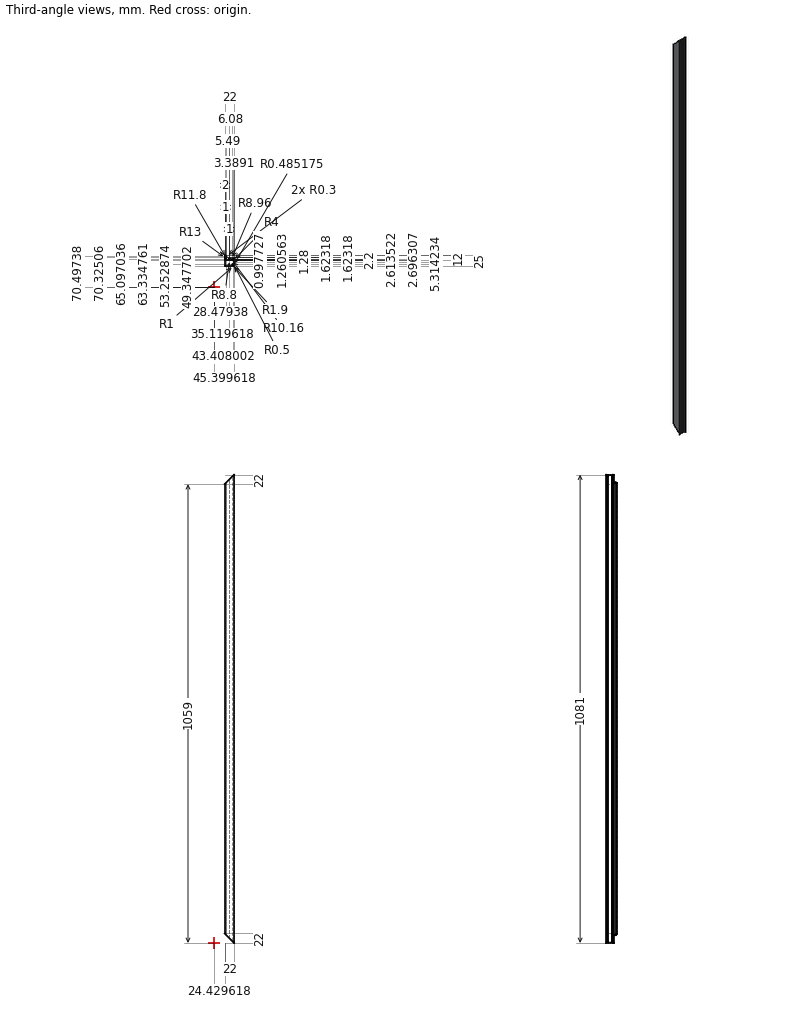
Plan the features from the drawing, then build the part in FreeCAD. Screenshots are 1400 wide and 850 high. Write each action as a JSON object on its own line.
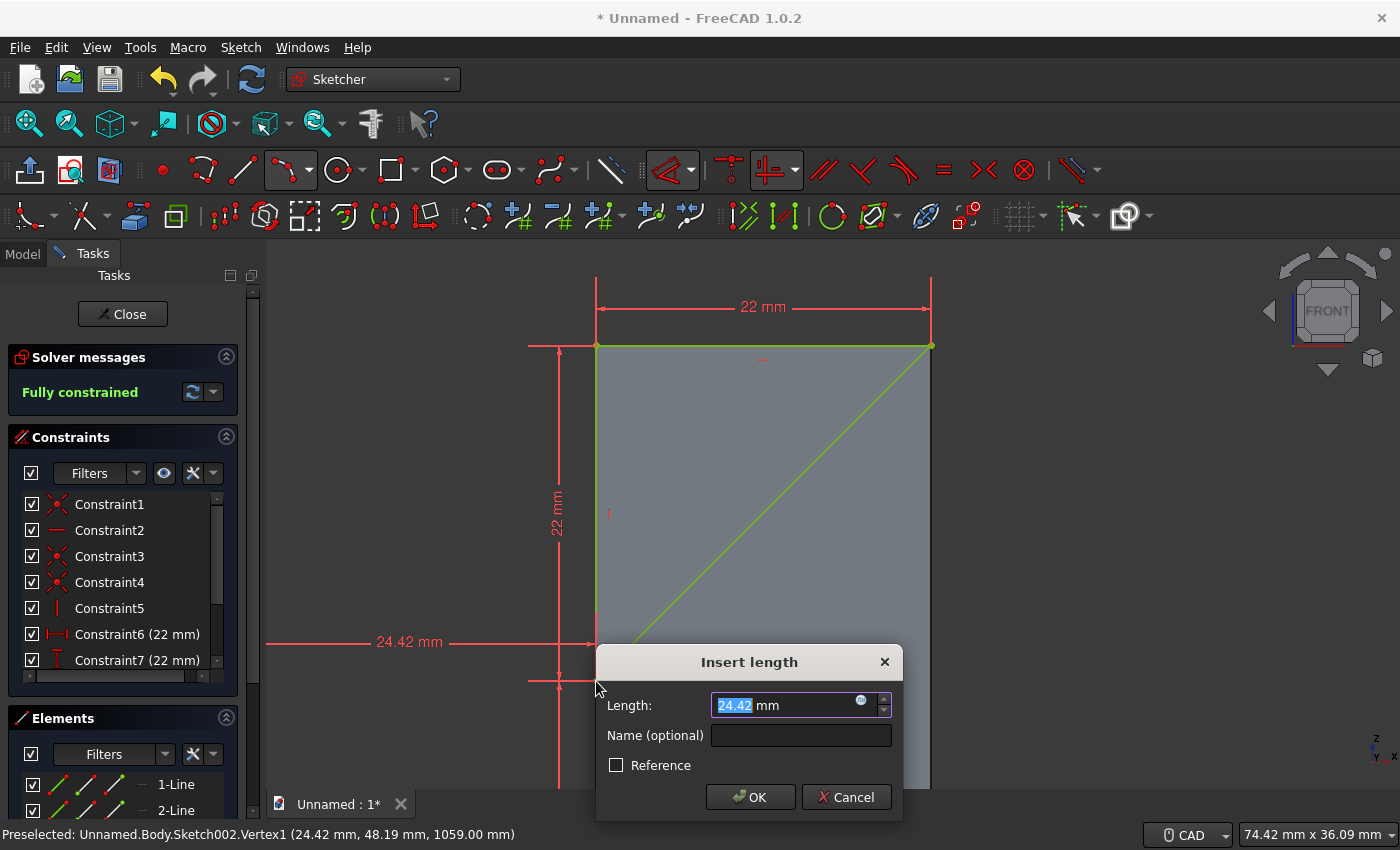
{"action": "type", "text": "24.429618"}
{"action": "key", "text": "Return"}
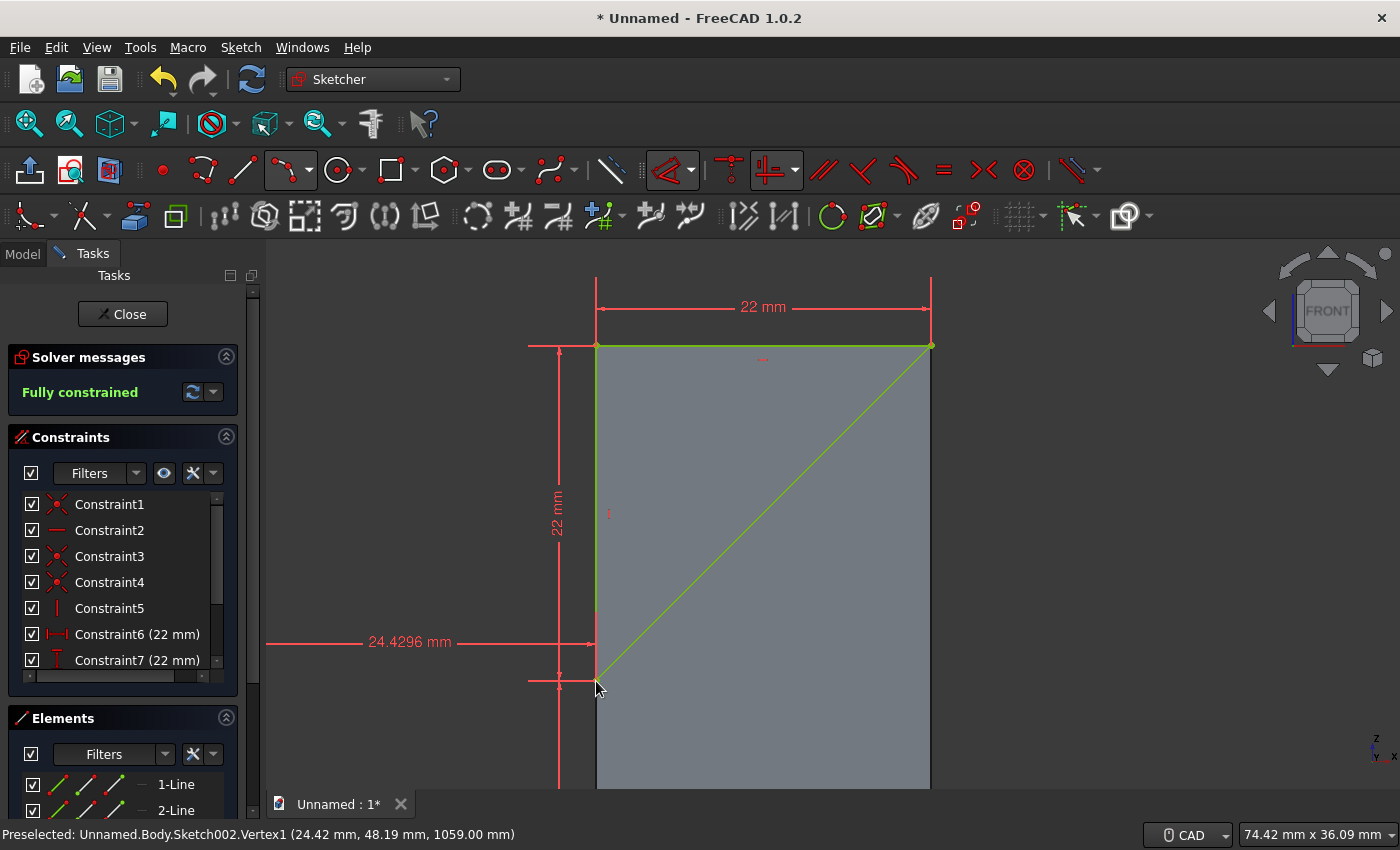
{"action": "left_click", "coordinate": [123, 314]}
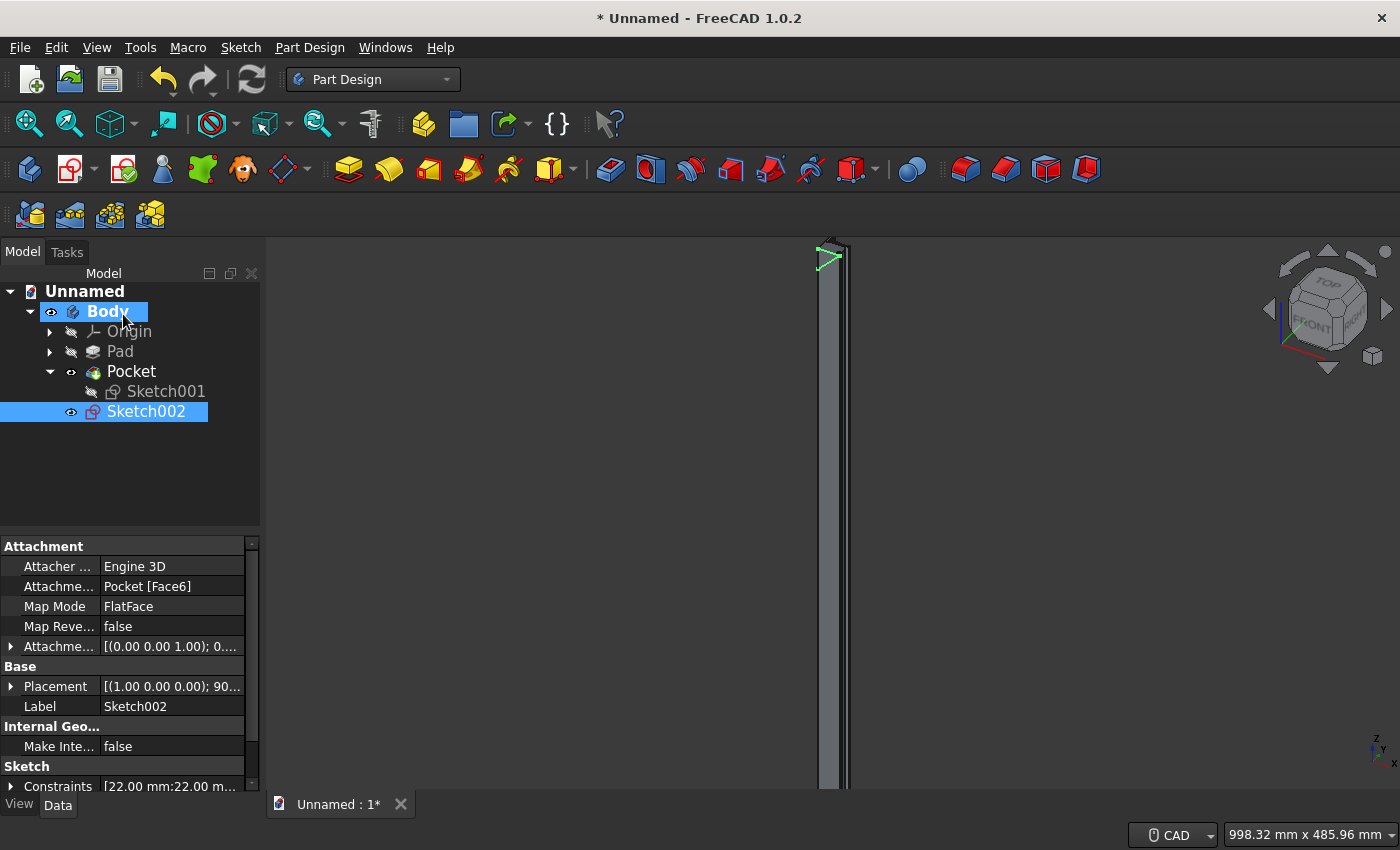
{"action": "left_click", "coordinate": [612, 170]}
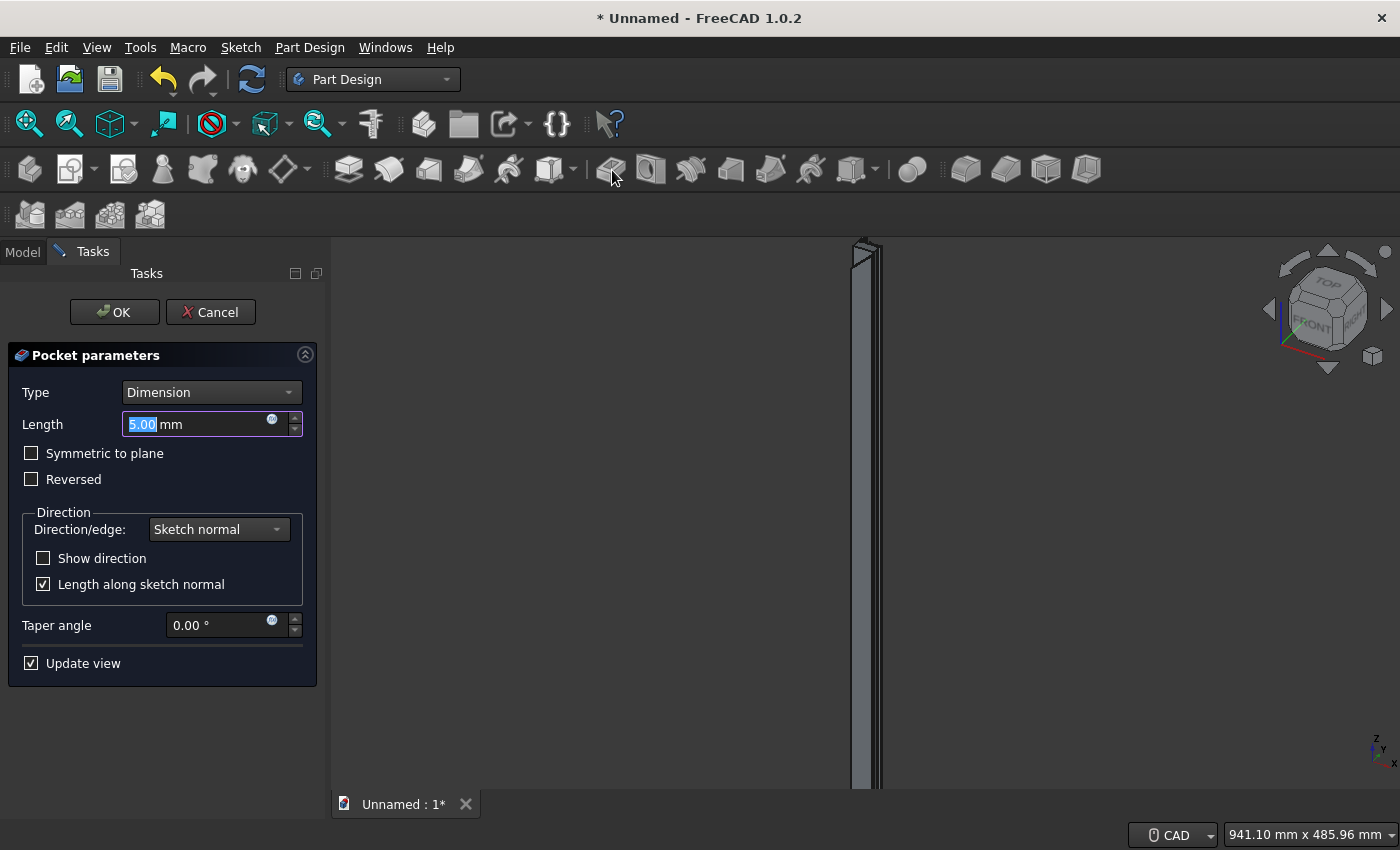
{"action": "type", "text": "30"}
{"action": "key", "text": "Tab"}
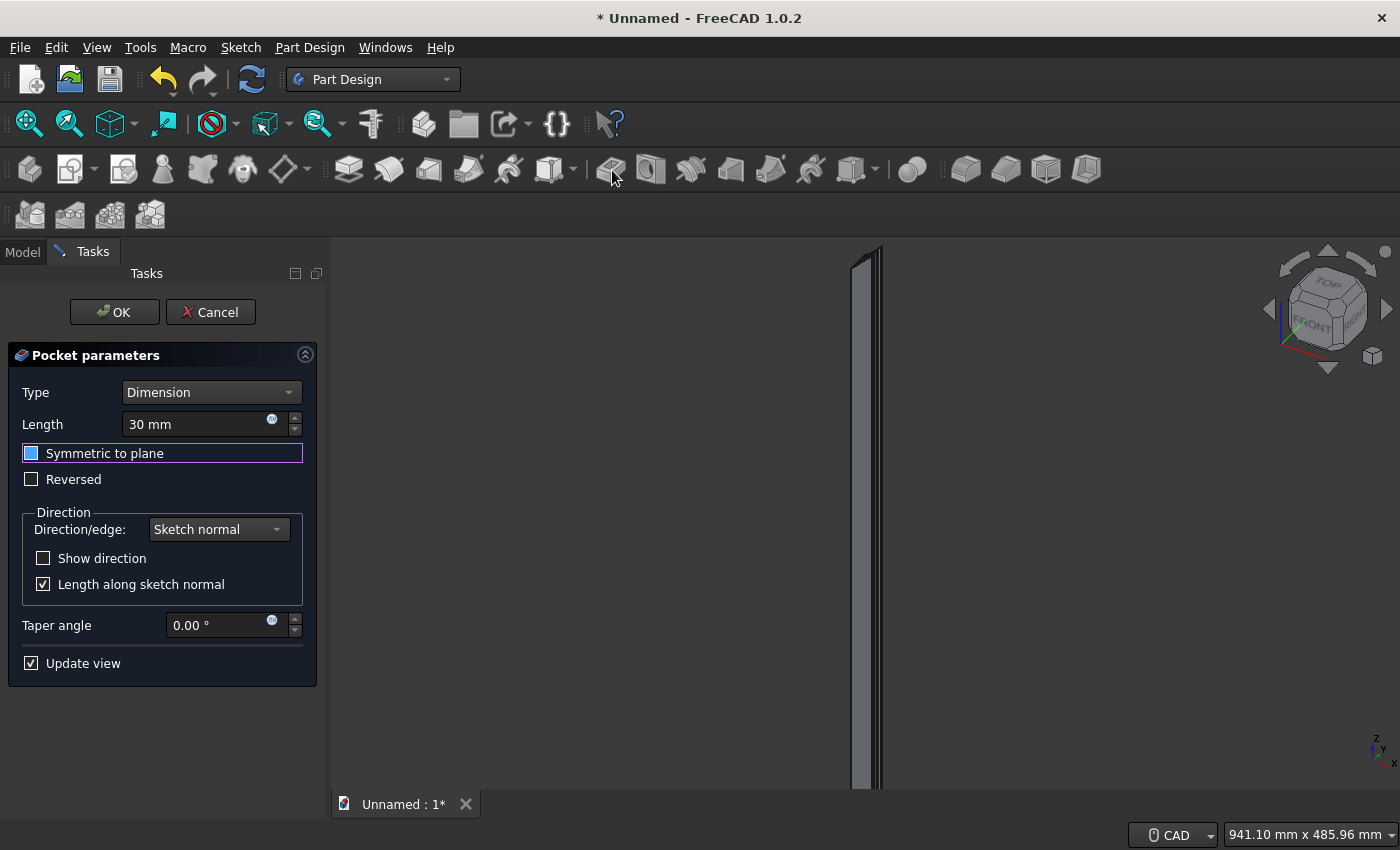
{"action": "left_click", "coordinate": [115, 312]}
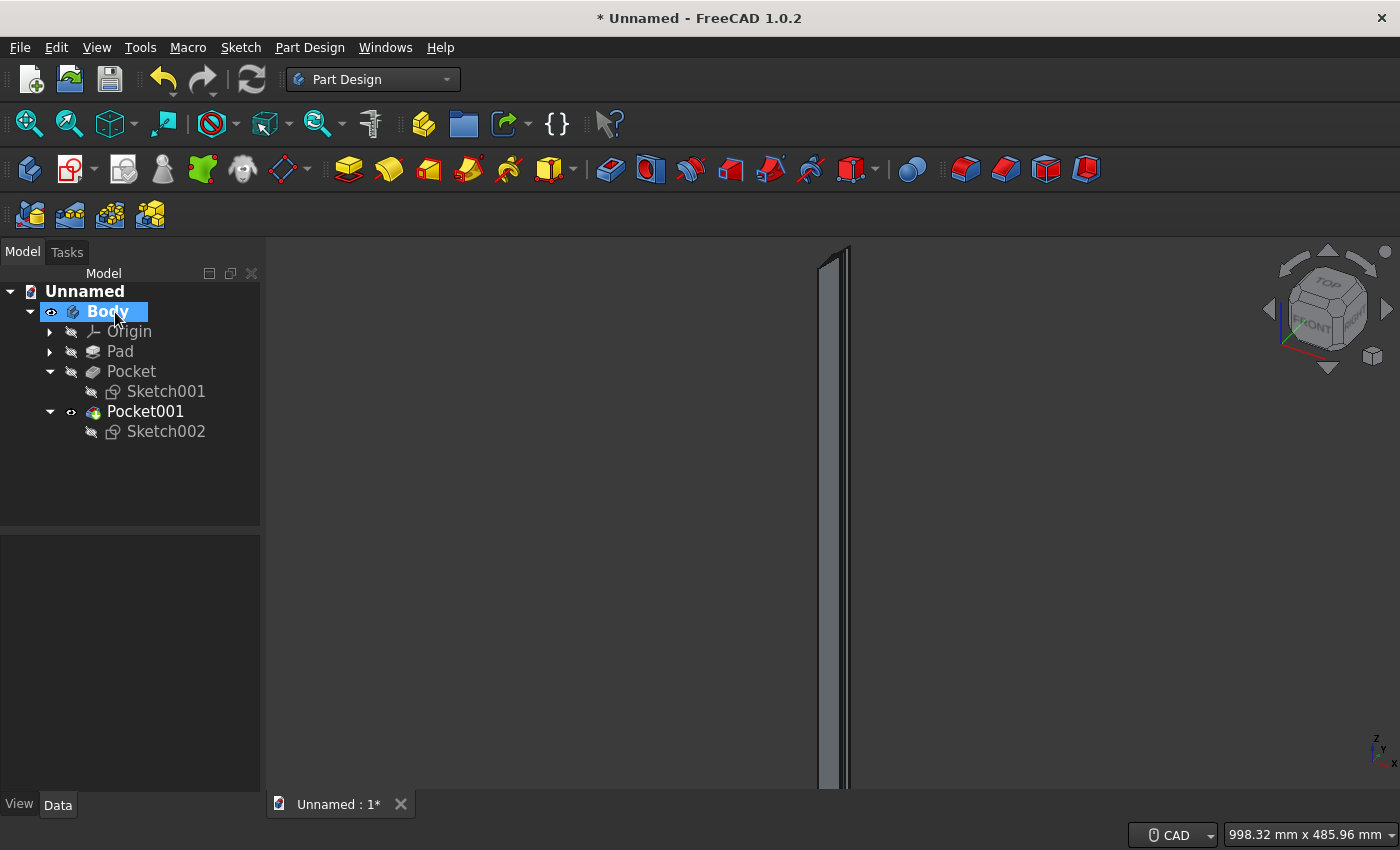
{"action": "key", "text": "0"}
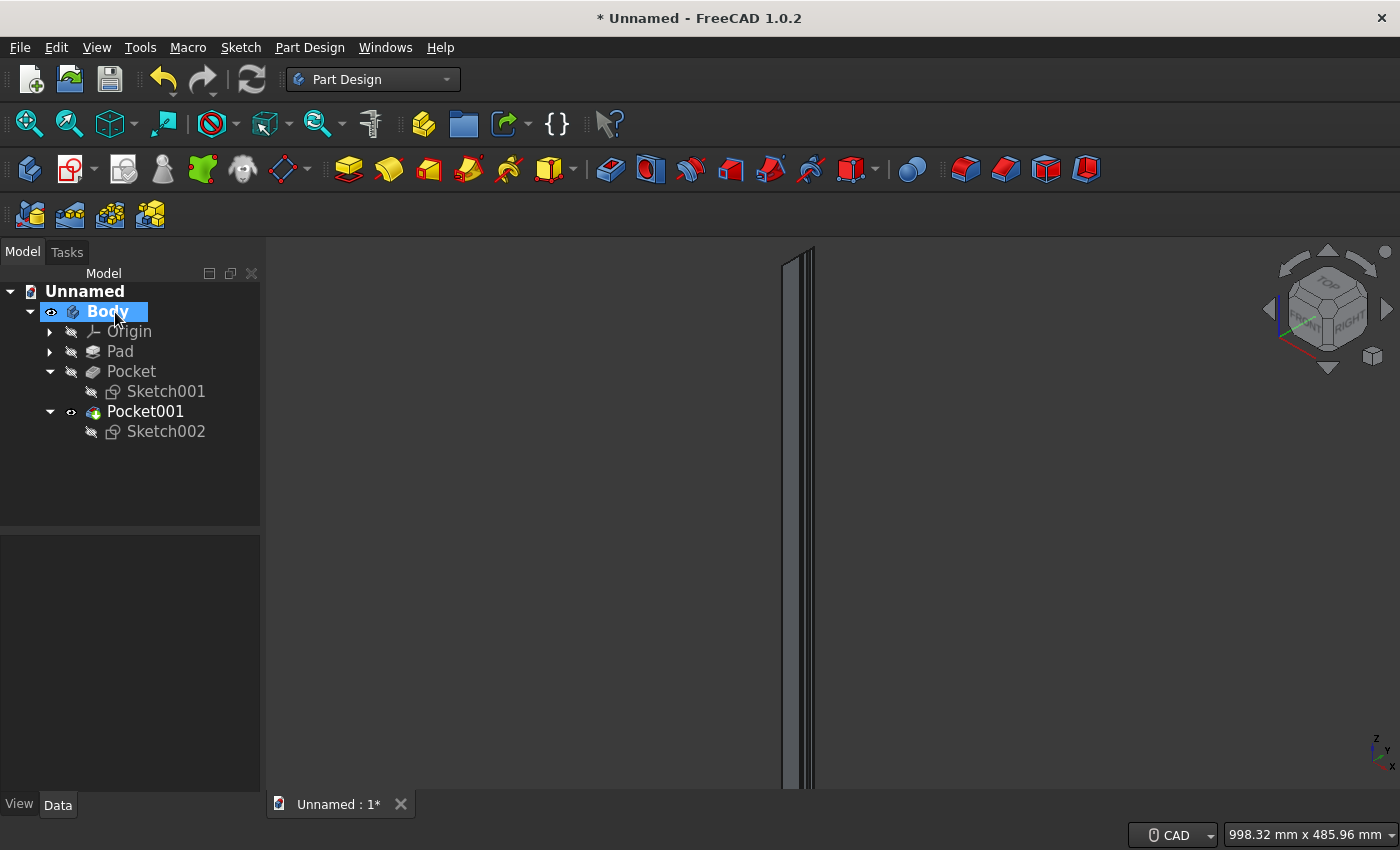
{"action": "left_click", "coordinate": [30, 124]}